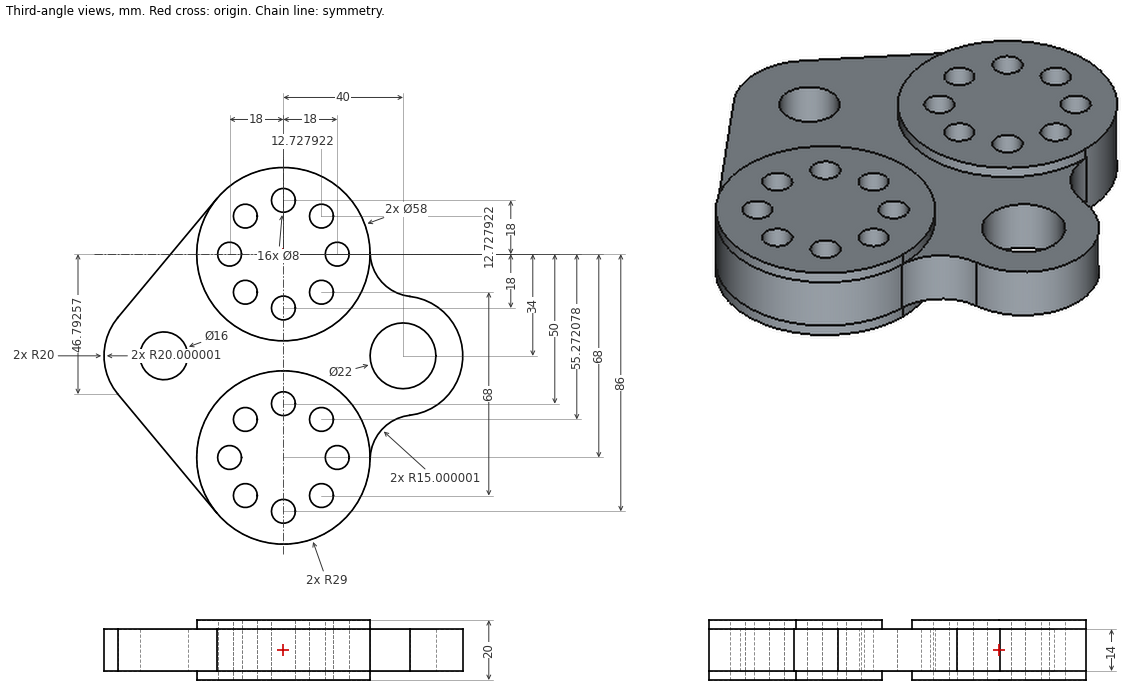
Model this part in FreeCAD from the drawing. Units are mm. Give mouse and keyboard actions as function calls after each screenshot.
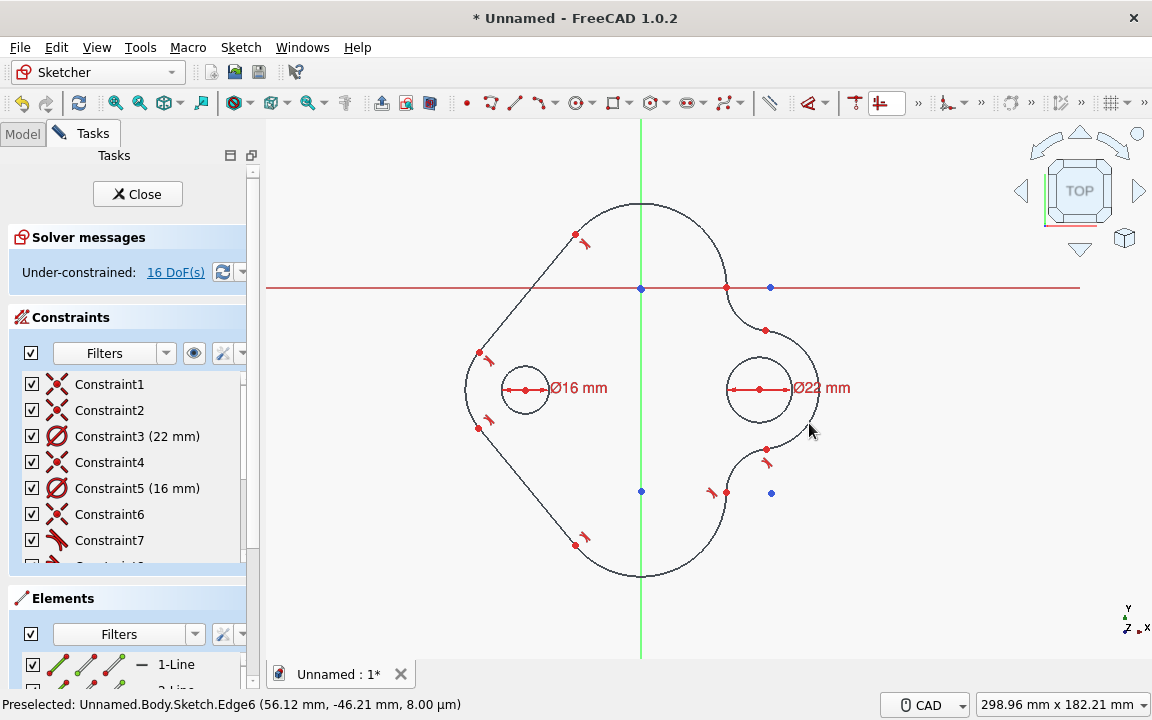
click(809, 423)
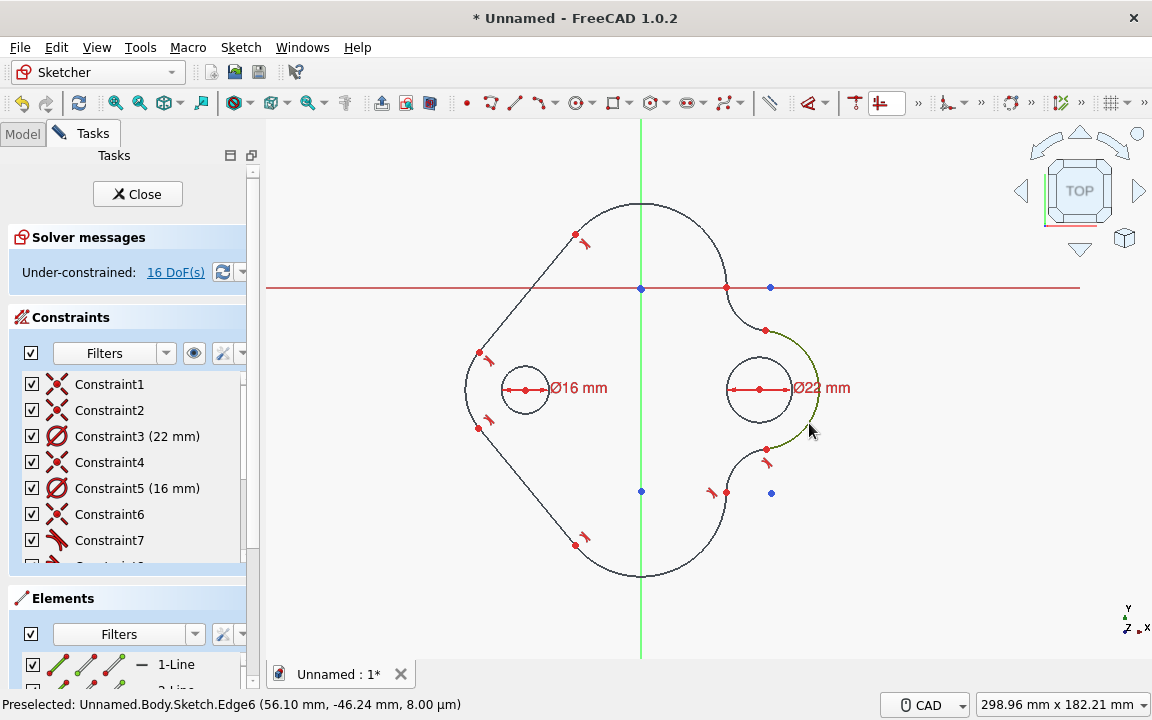
click(731, 306)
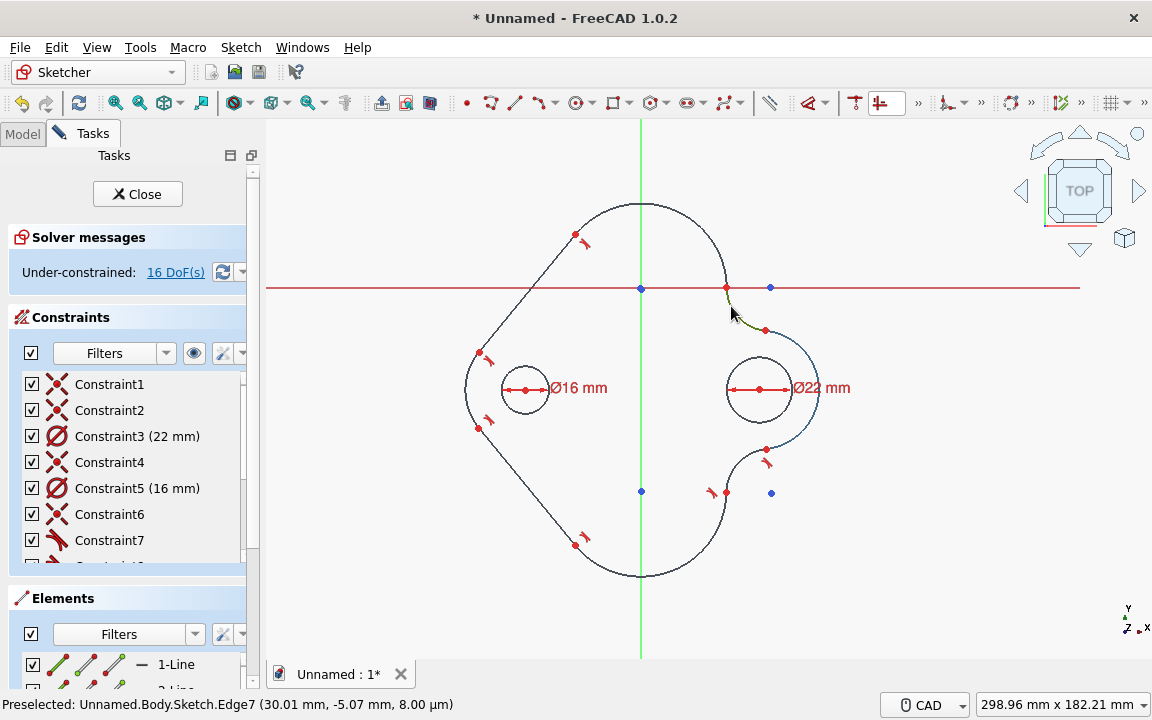
key(t)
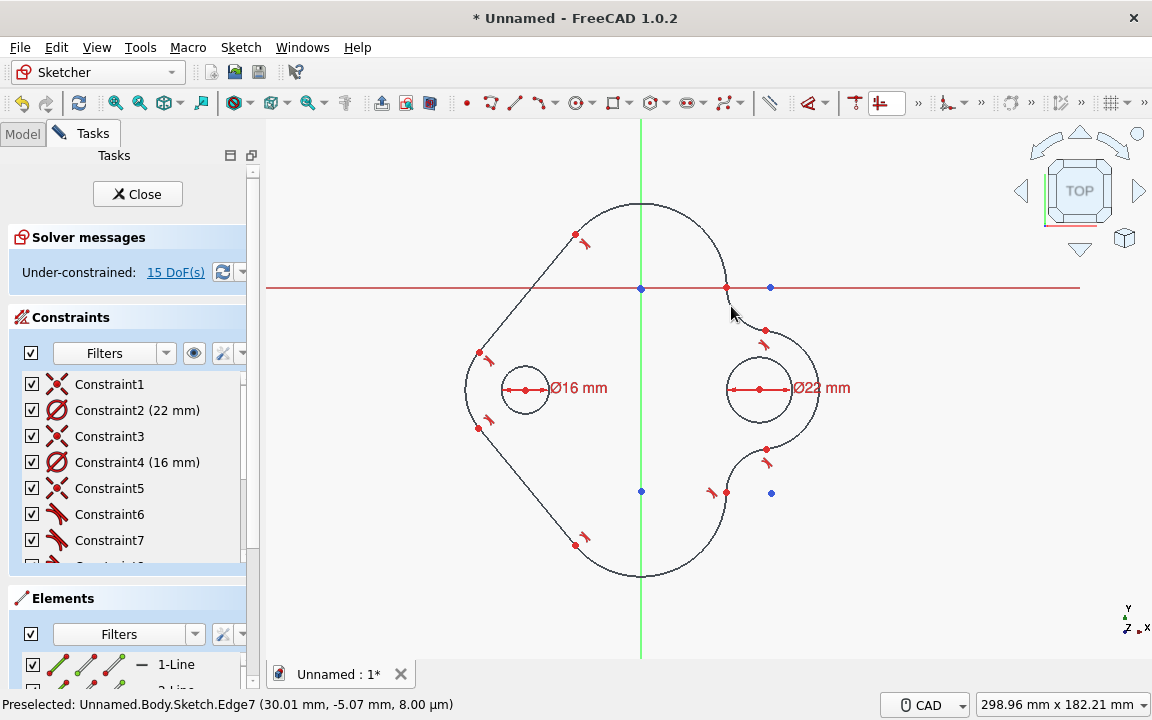
click(731, 306)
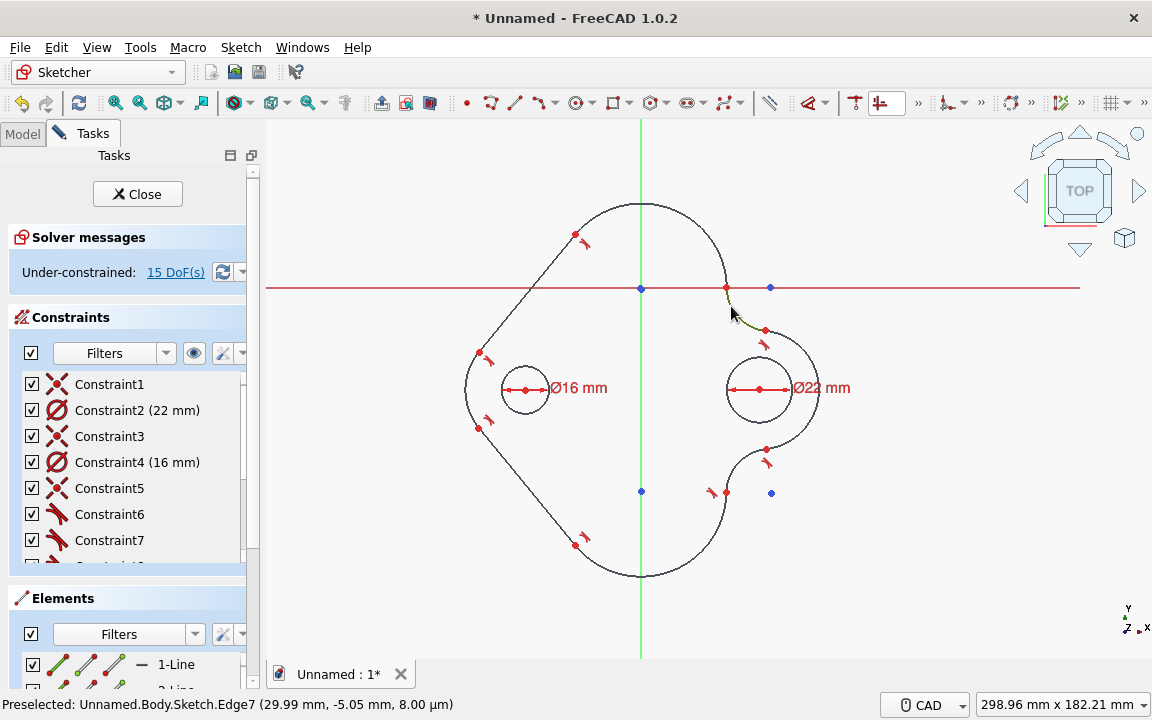
click(704, 231)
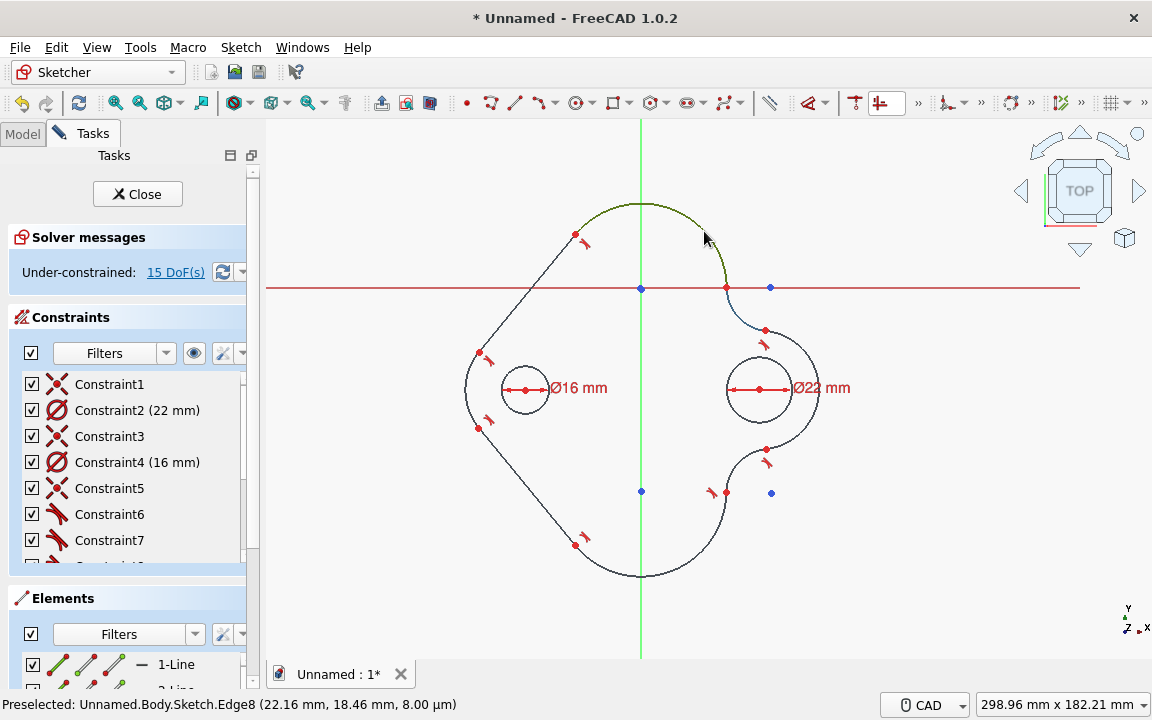
key(t)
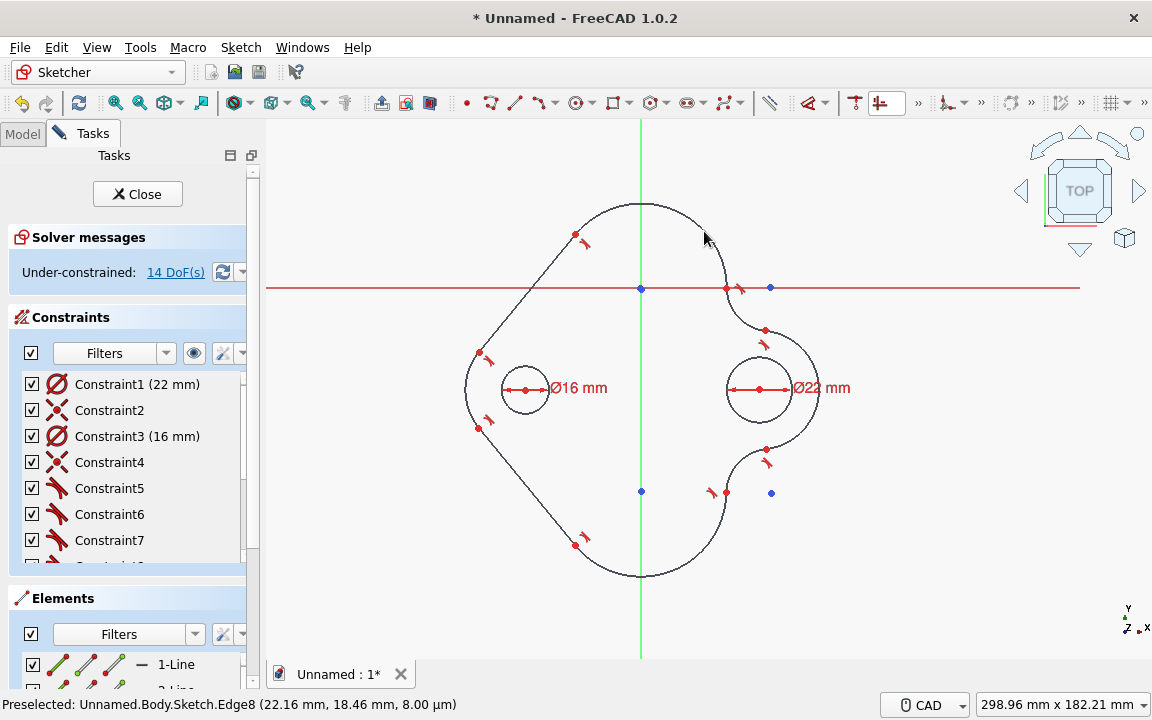
scroll(641, 289, up, 3)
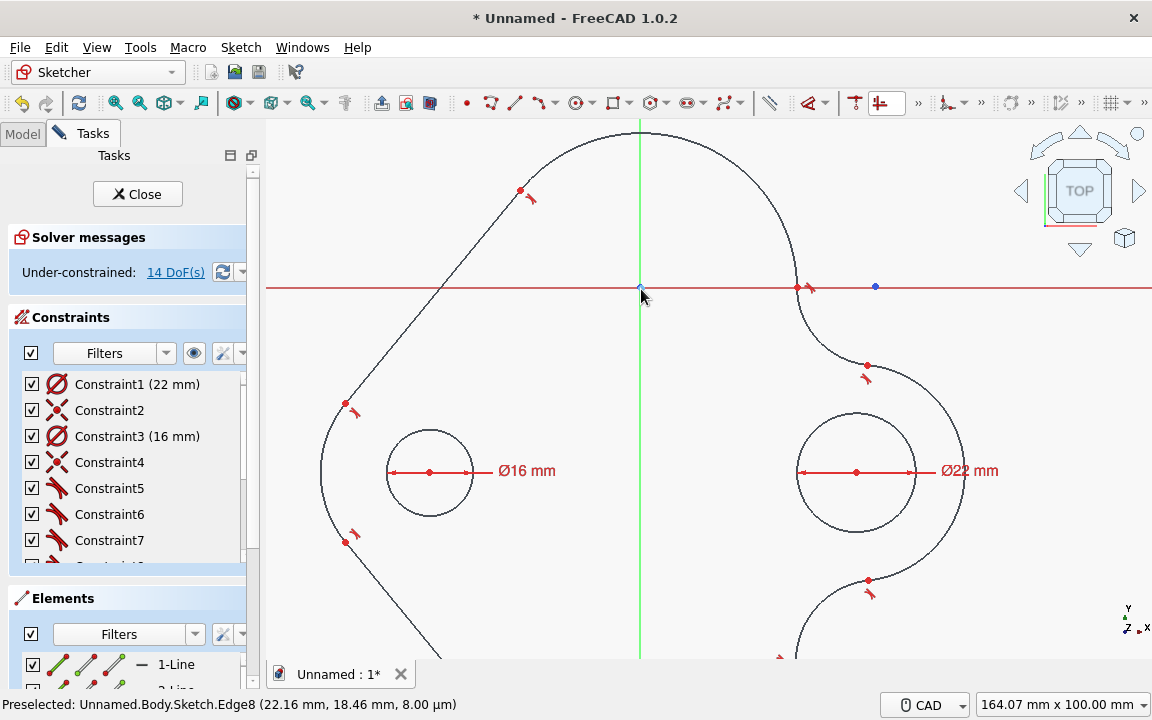
drag(630, 278, 651, 299)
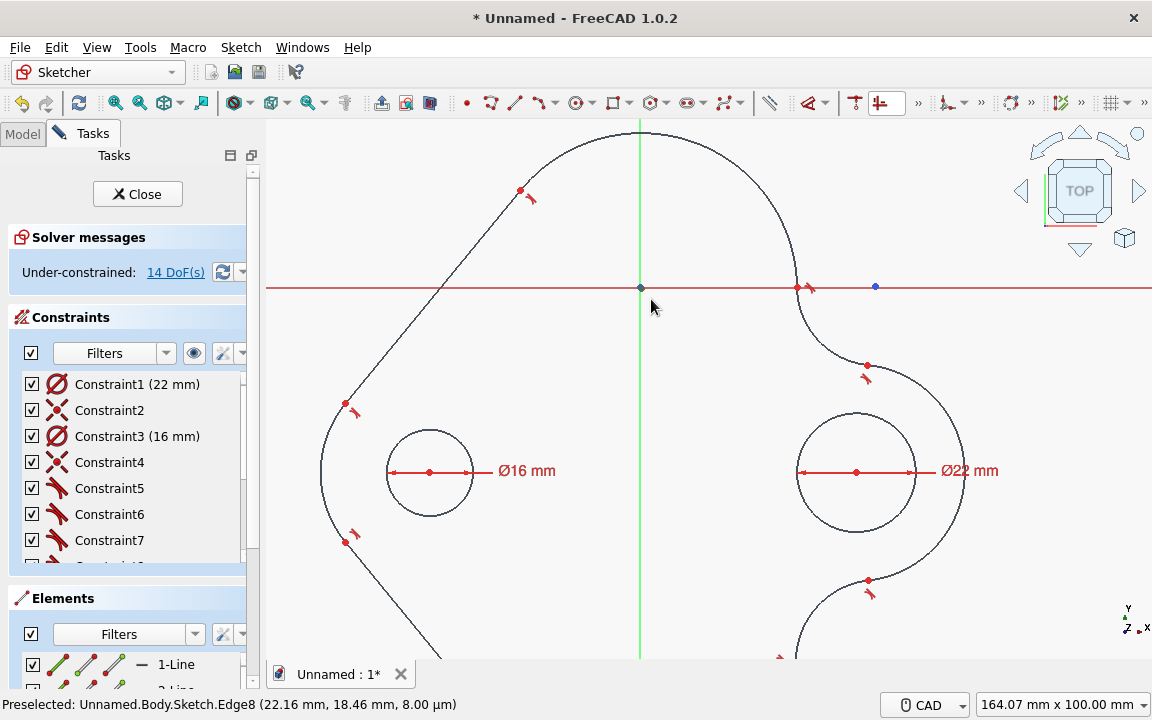
key(c)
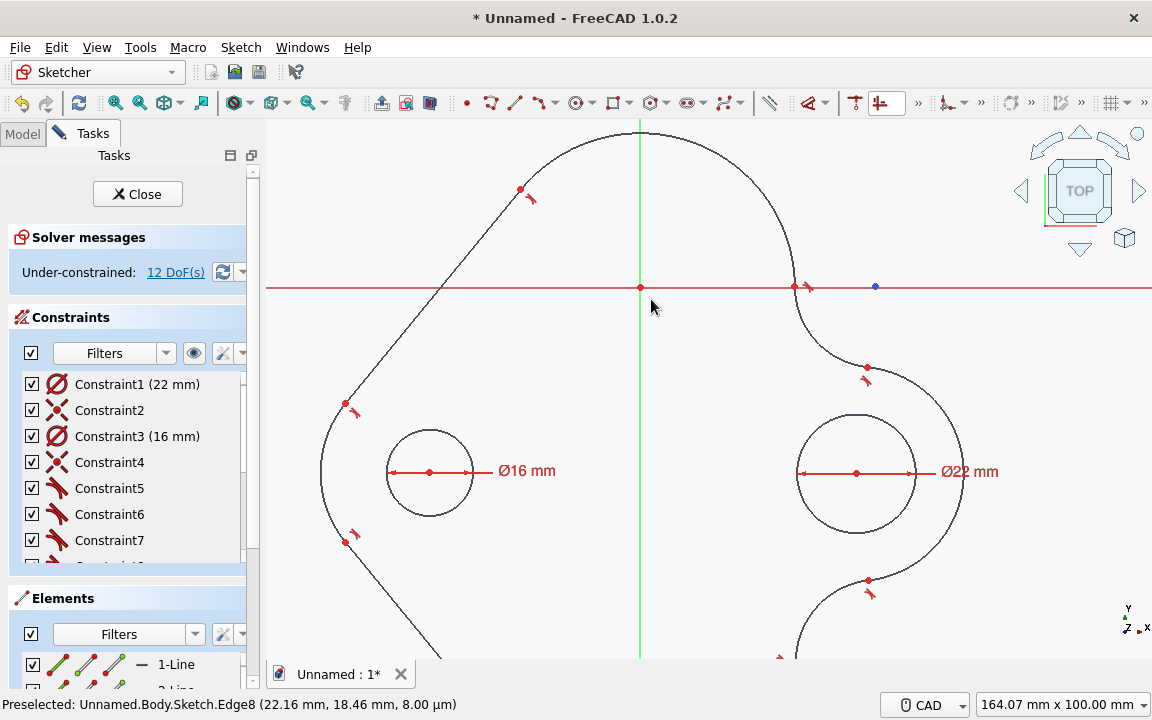
click(835, 592)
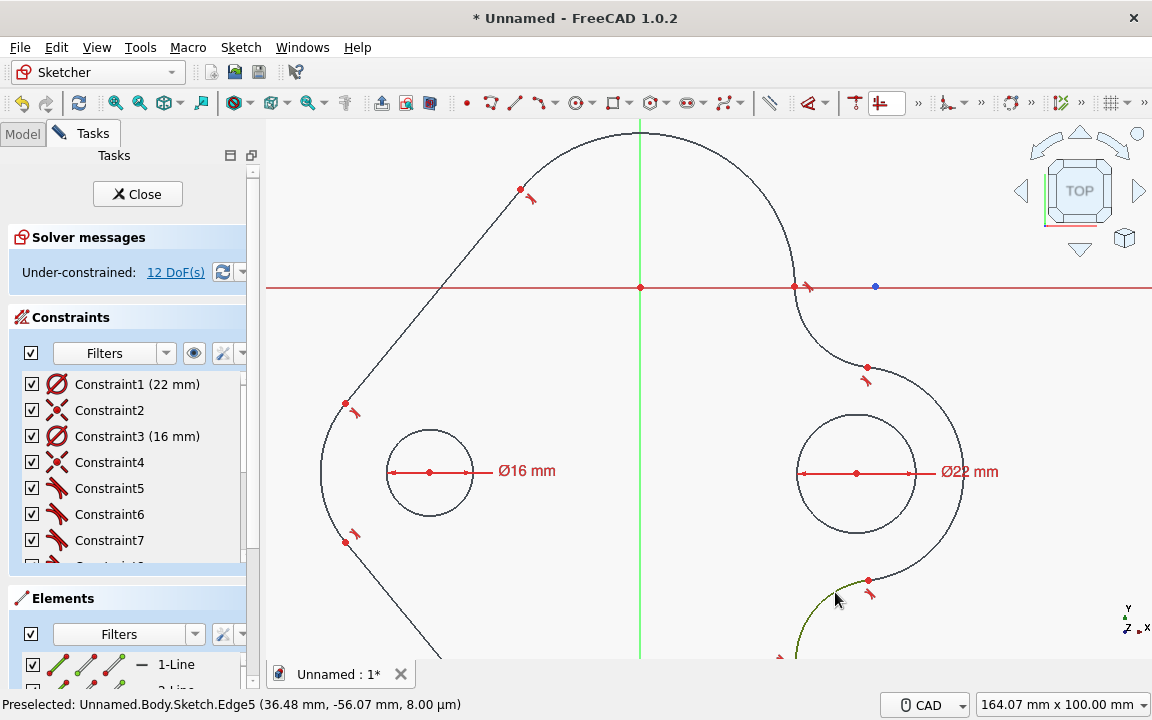
click(803, 321)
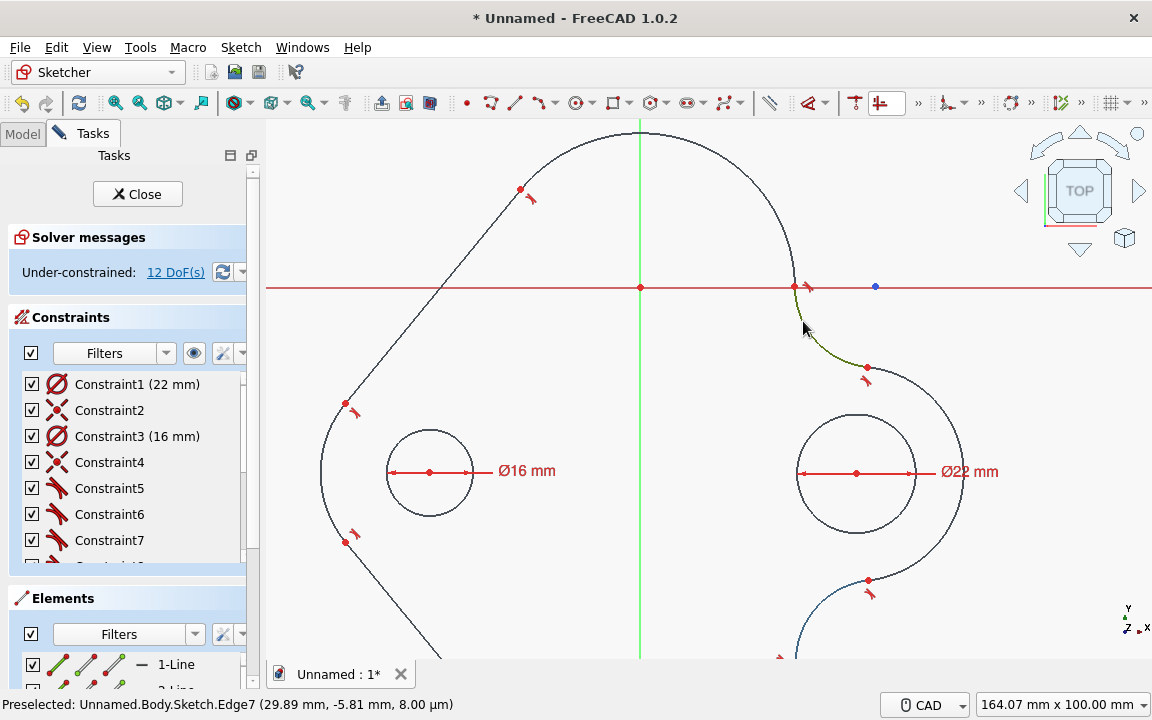
key(e)